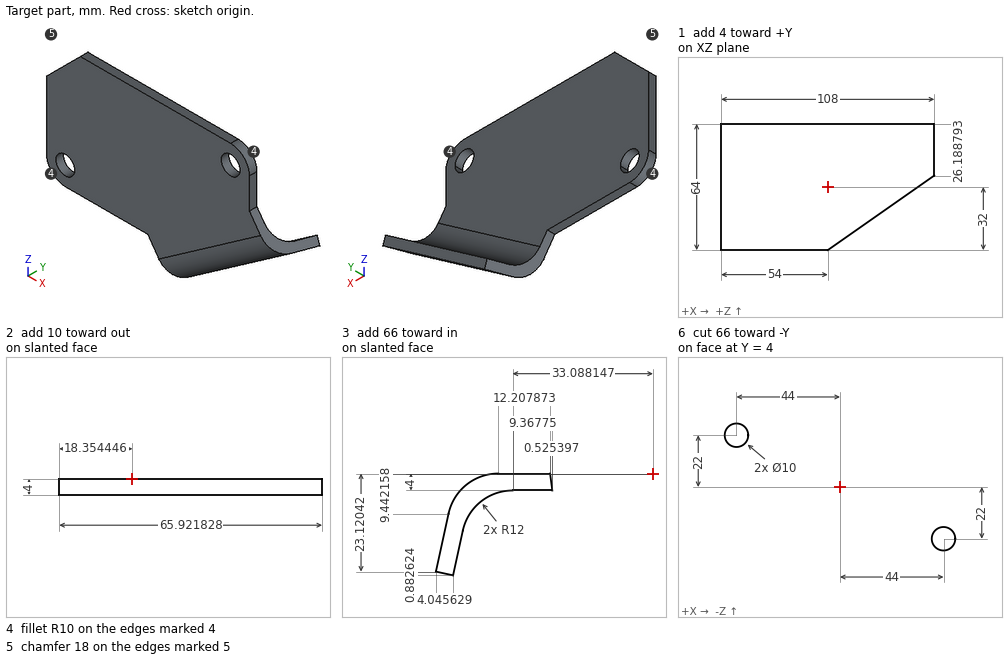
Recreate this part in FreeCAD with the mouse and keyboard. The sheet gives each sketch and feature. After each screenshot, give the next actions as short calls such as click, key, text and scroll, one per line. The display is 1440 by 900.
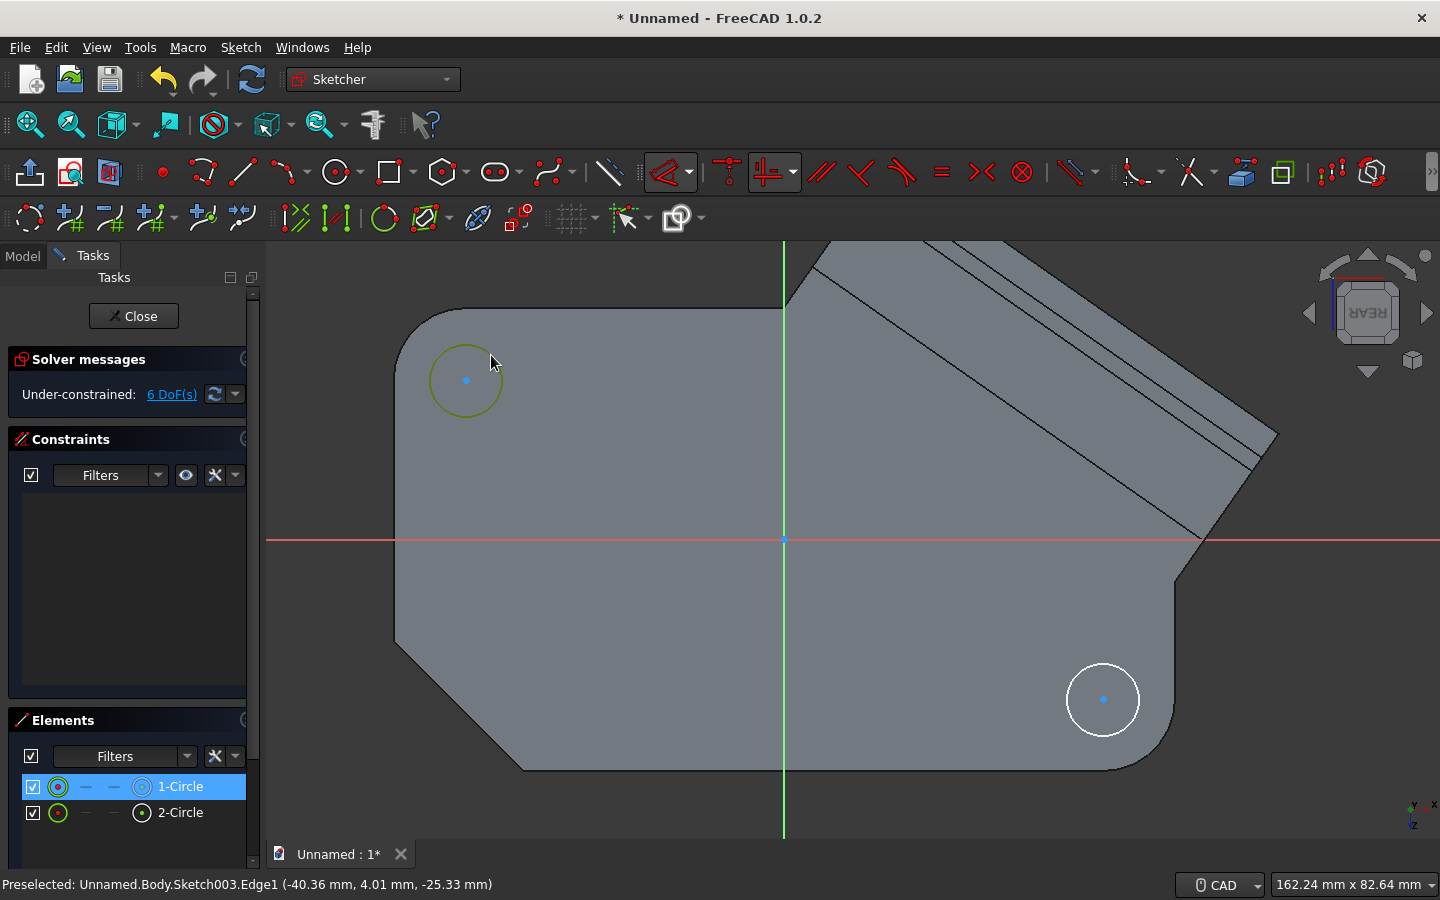
click(1128, 674)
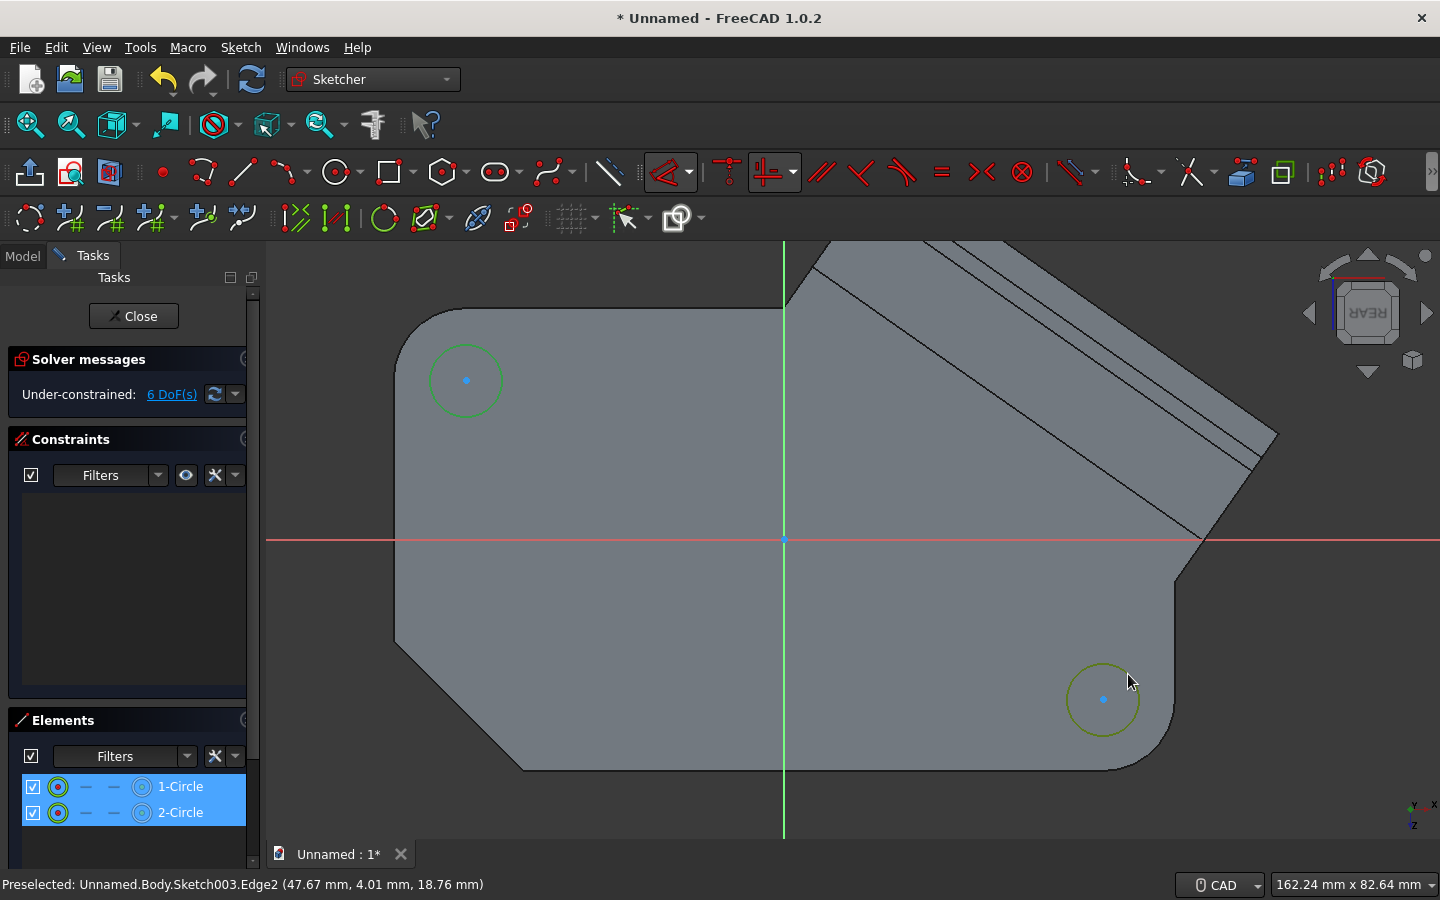
click(942, 172)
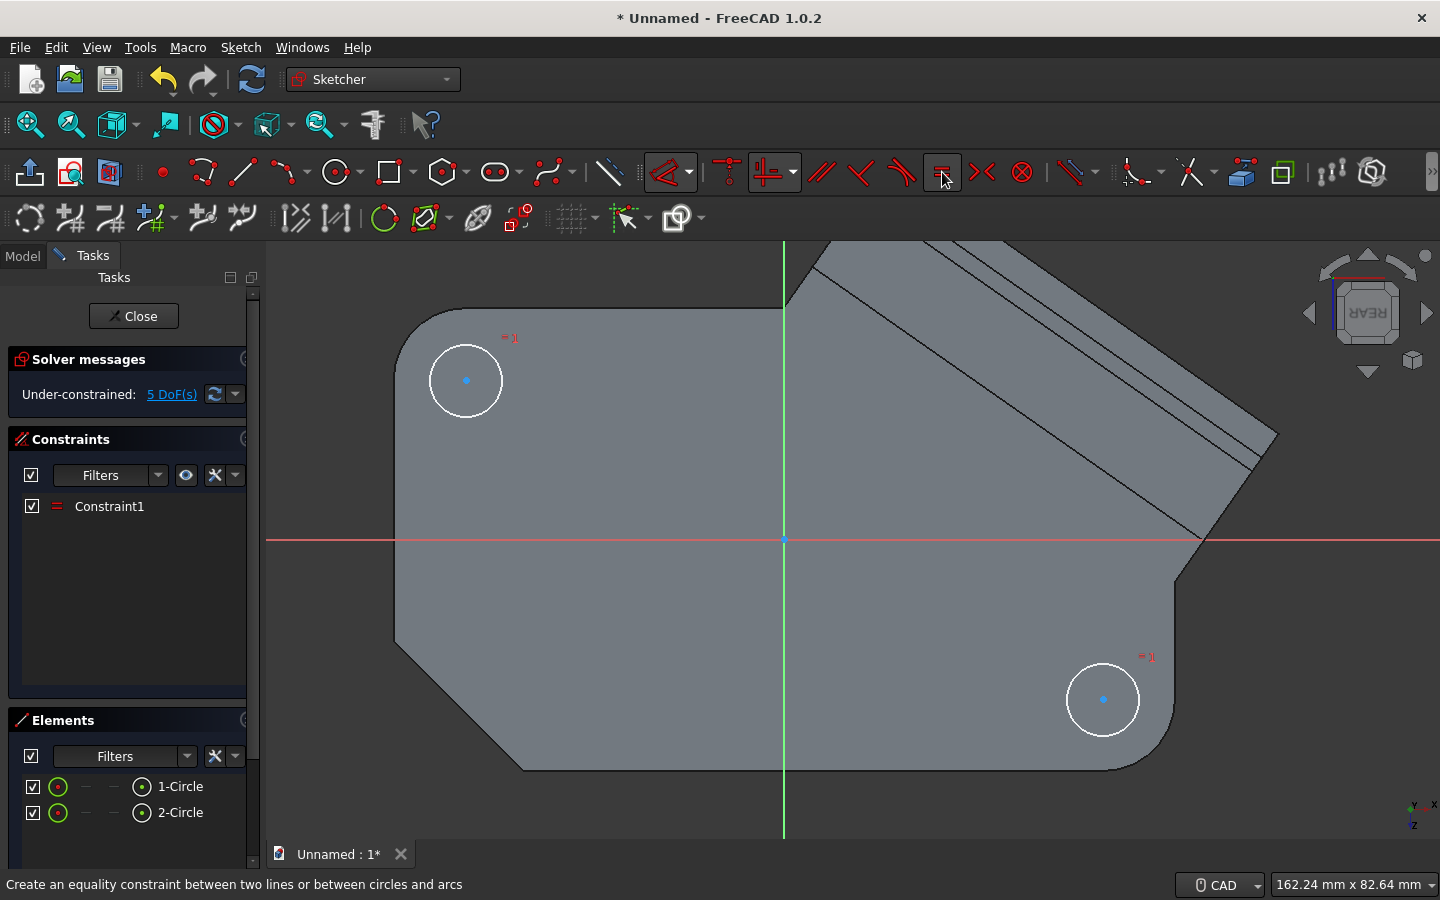
click(491, 355)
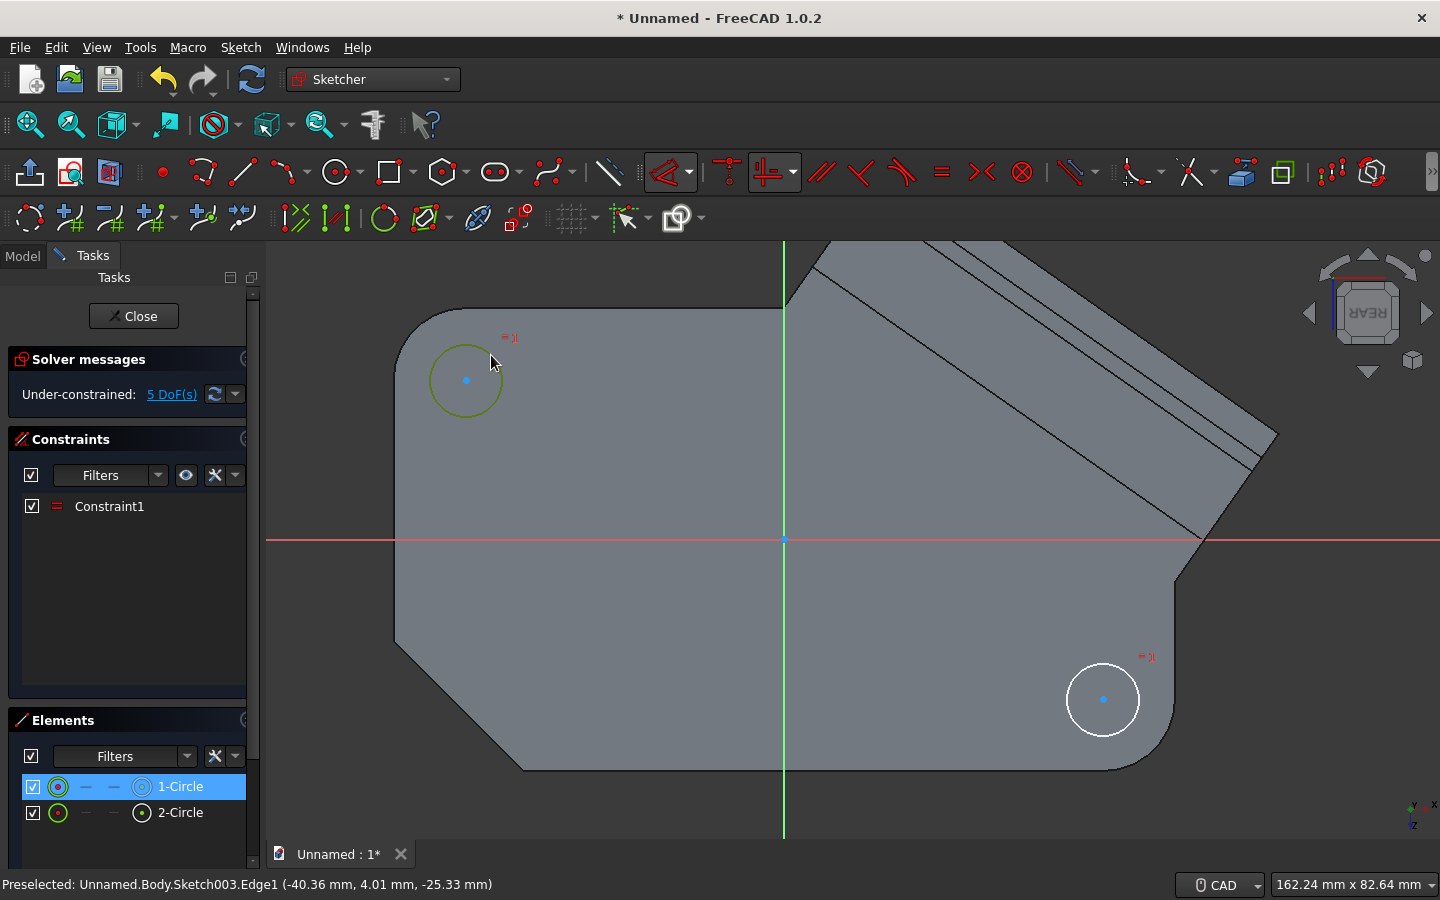
key(k)
key(o)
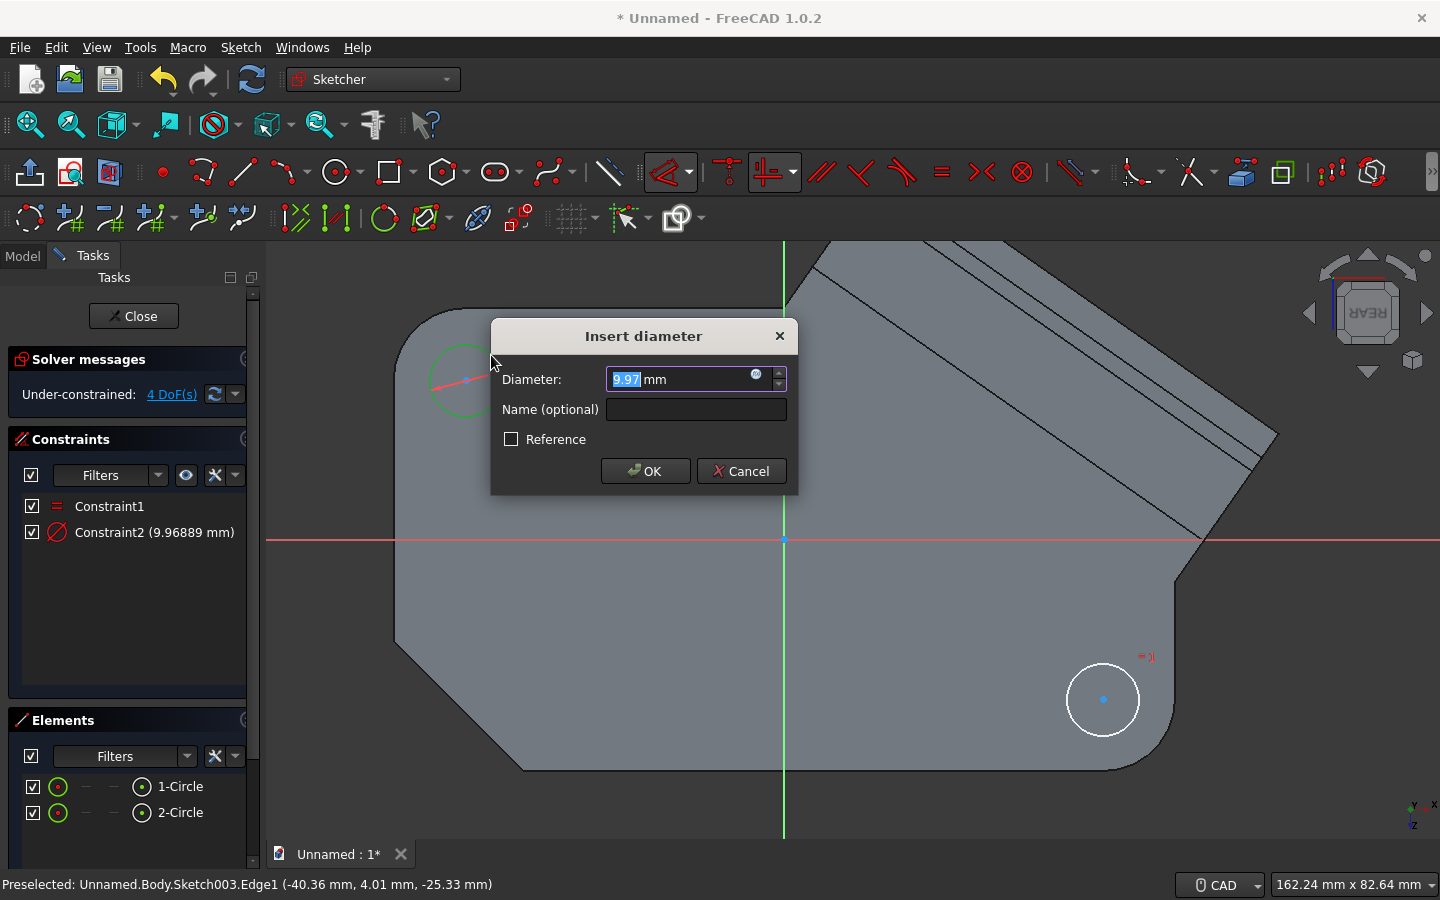
text(10)
key(Return)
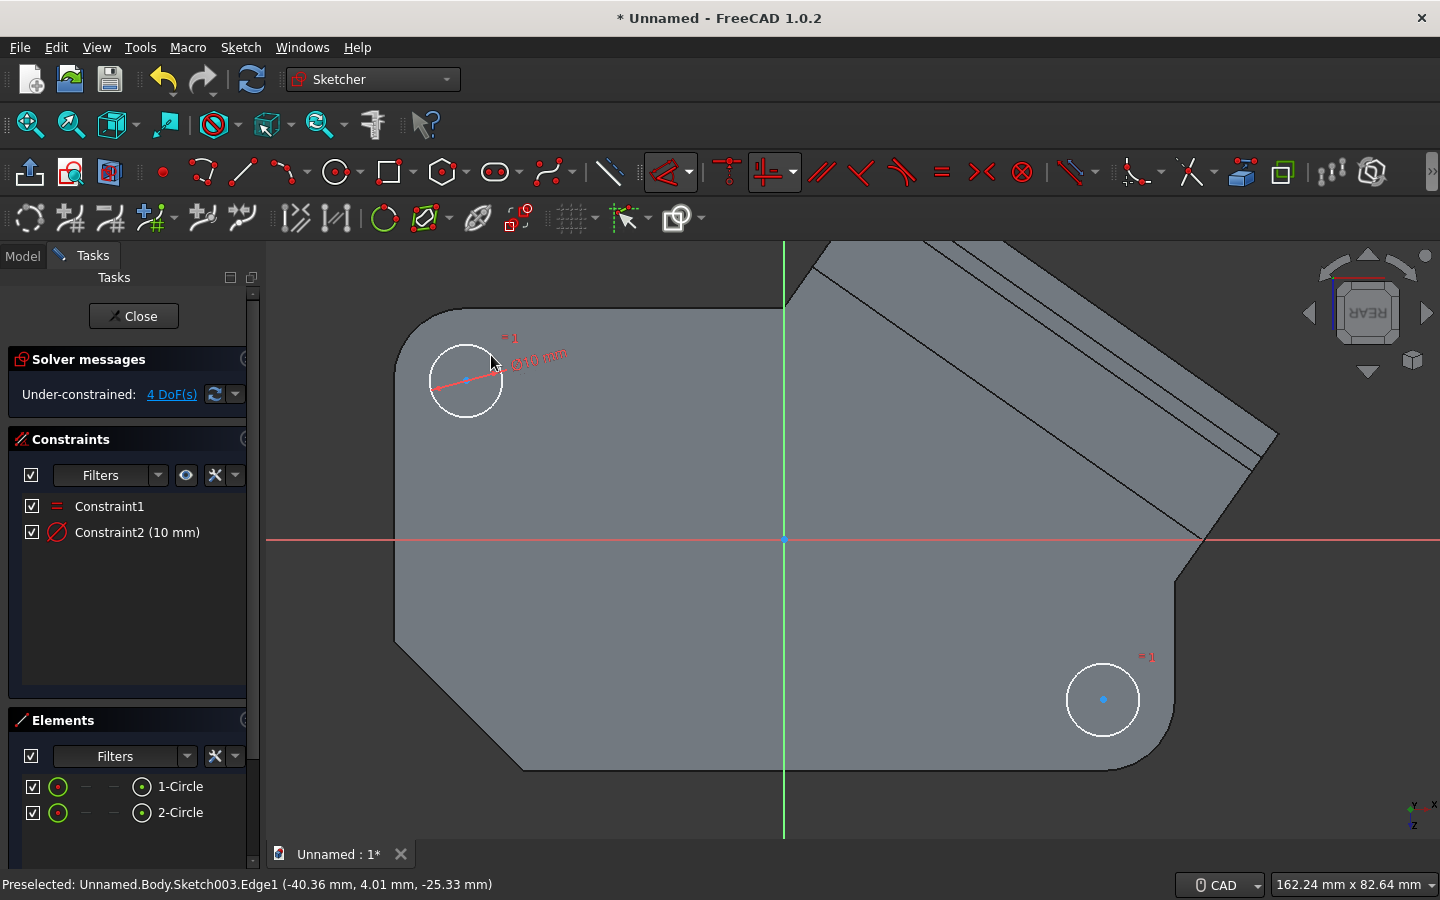
click(466, 381)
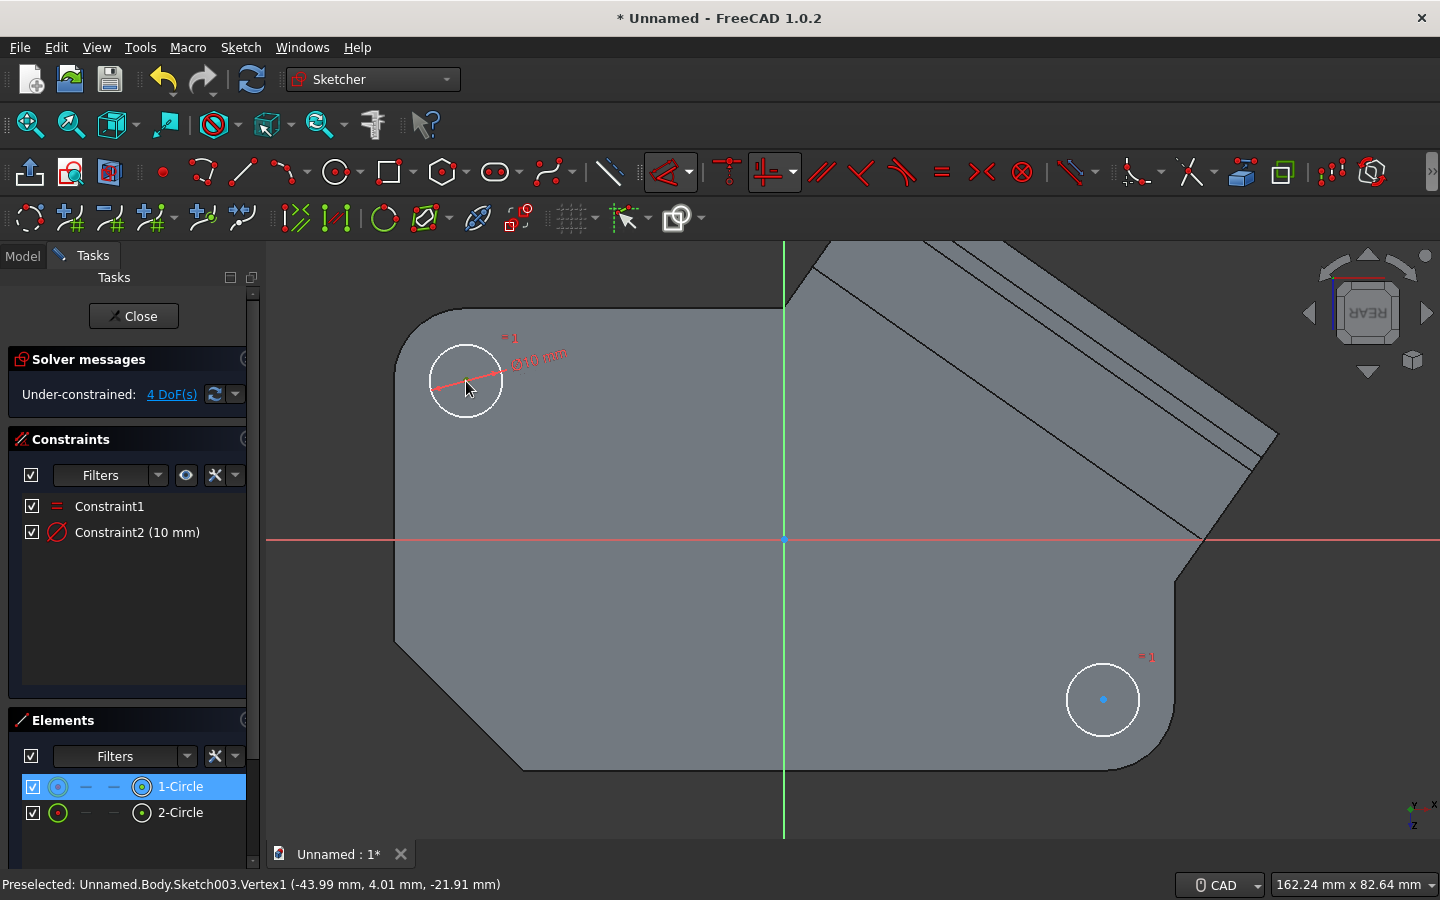
key(l)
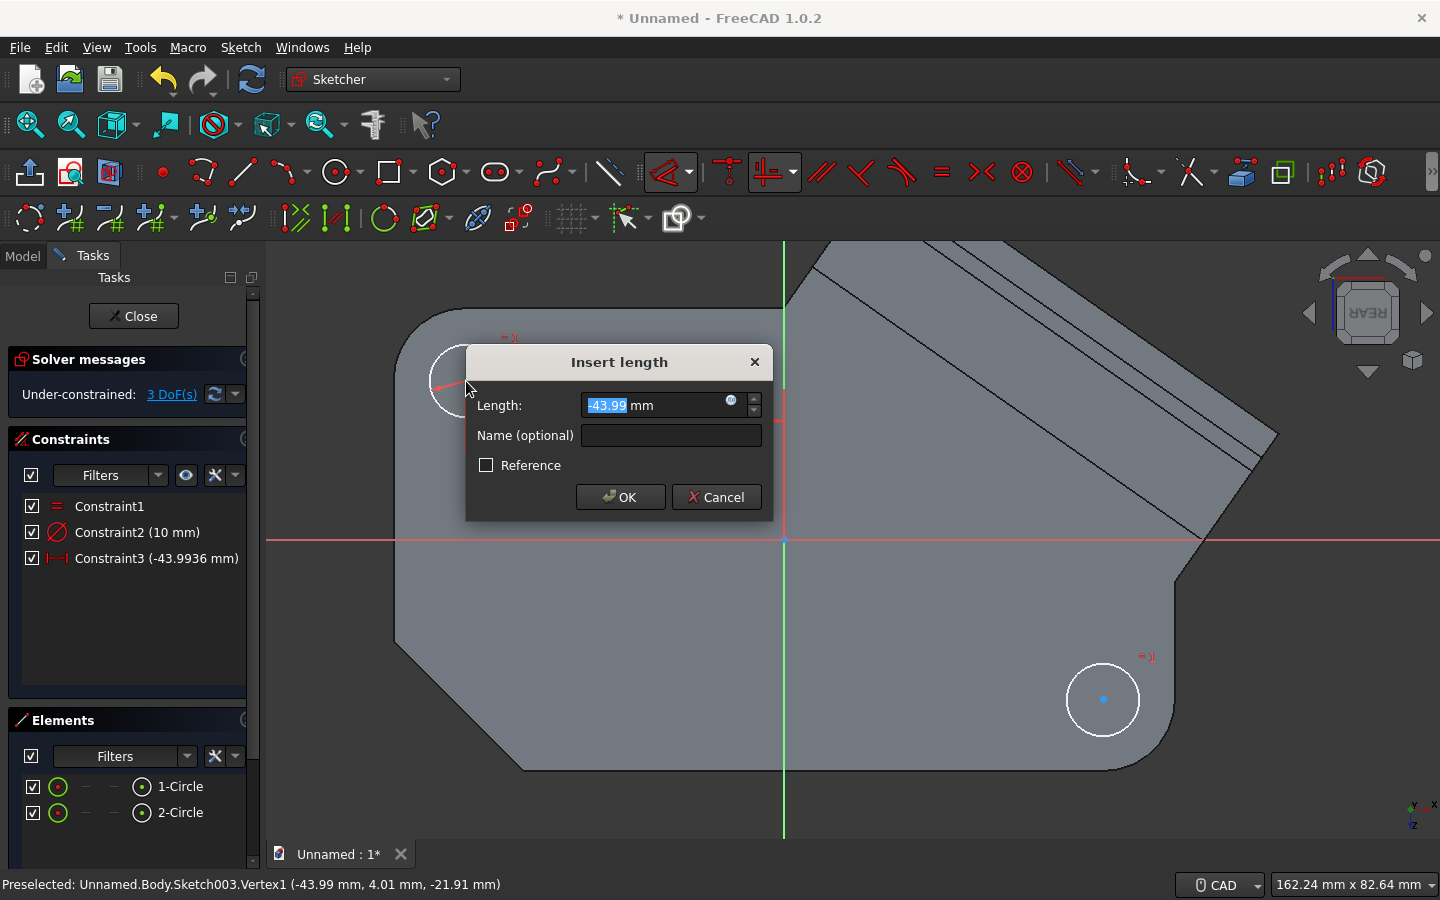
text(-44)
key(Return)